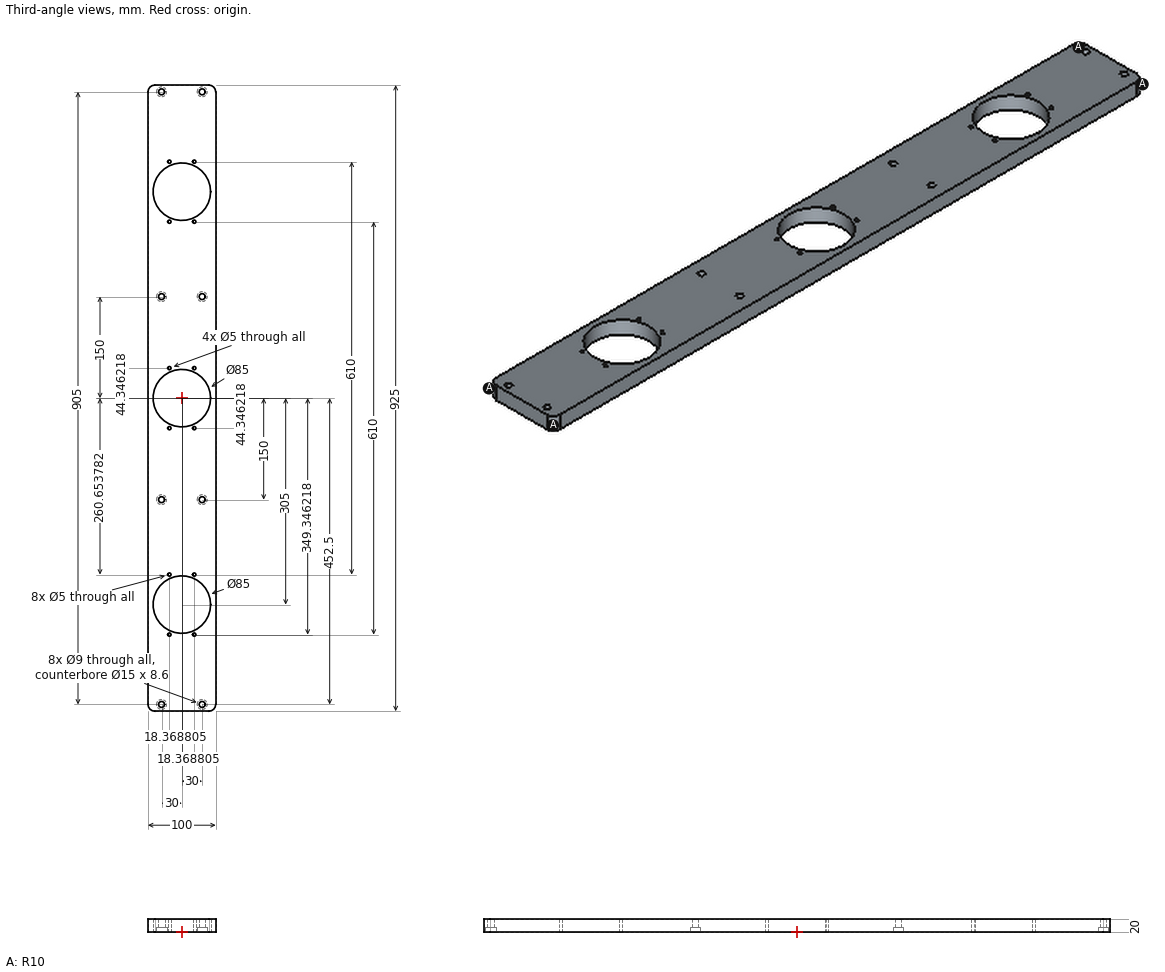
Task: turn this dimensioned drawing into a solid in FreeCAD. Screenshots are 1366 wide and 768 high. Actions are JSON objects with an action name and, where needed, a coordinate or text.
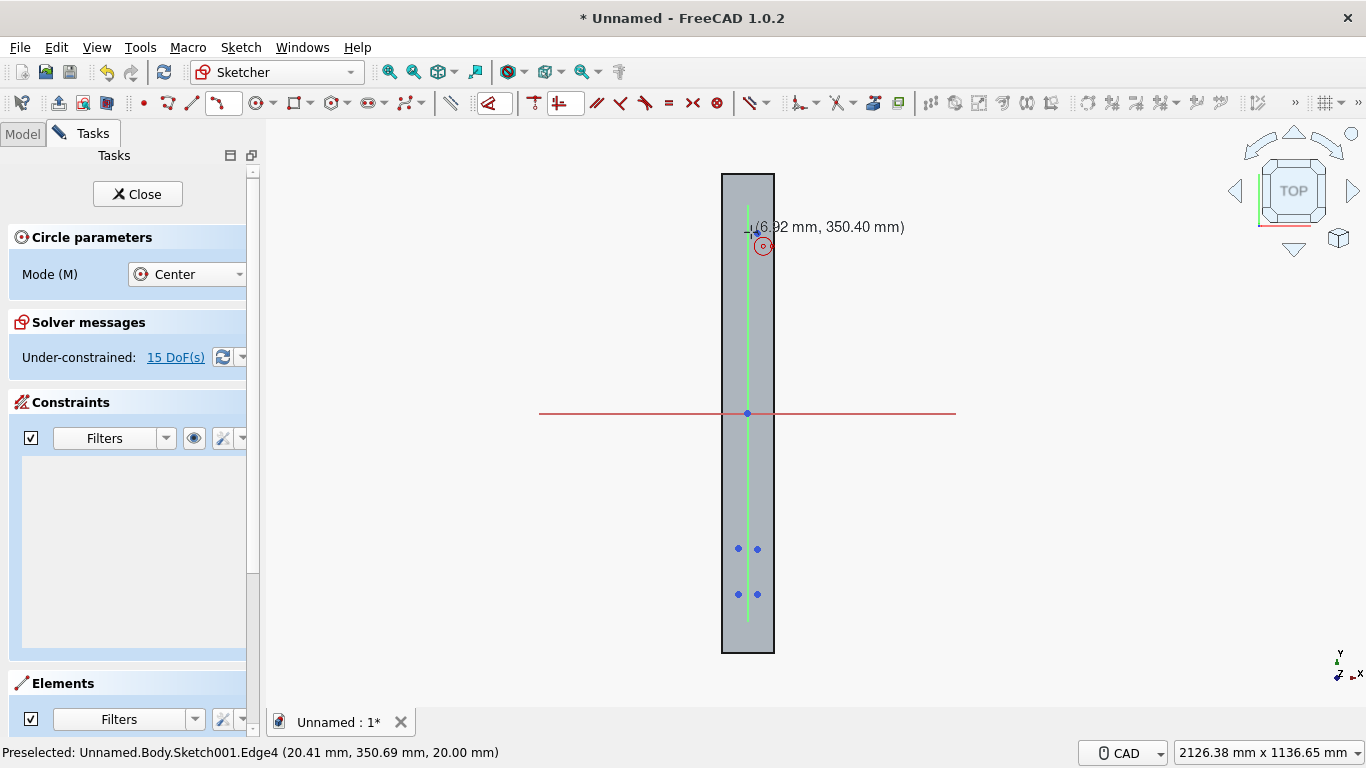
{"action": "scroll", "coordinate": [738, 233], "scroll_direction": "up", "scroll_amount": 3}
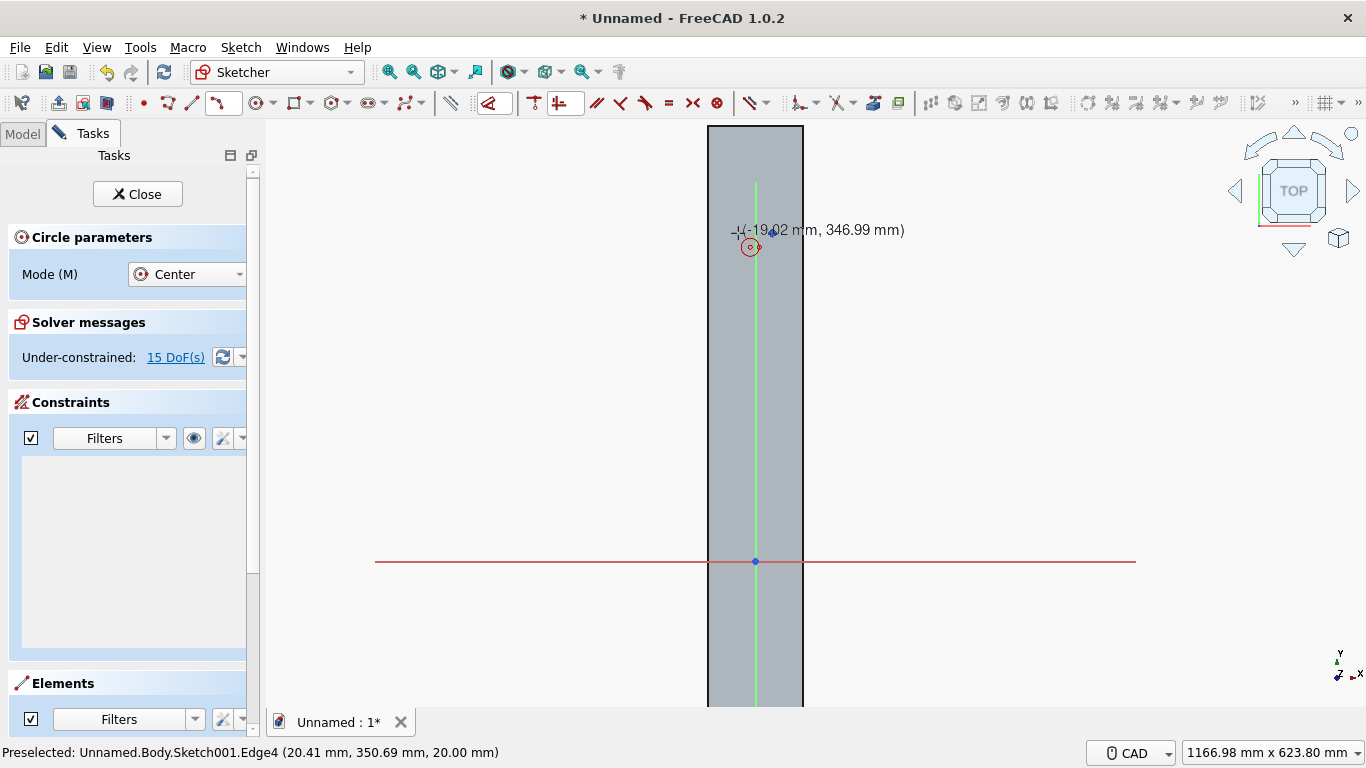
{"action": "left_click", "coordinate": [738, 232]}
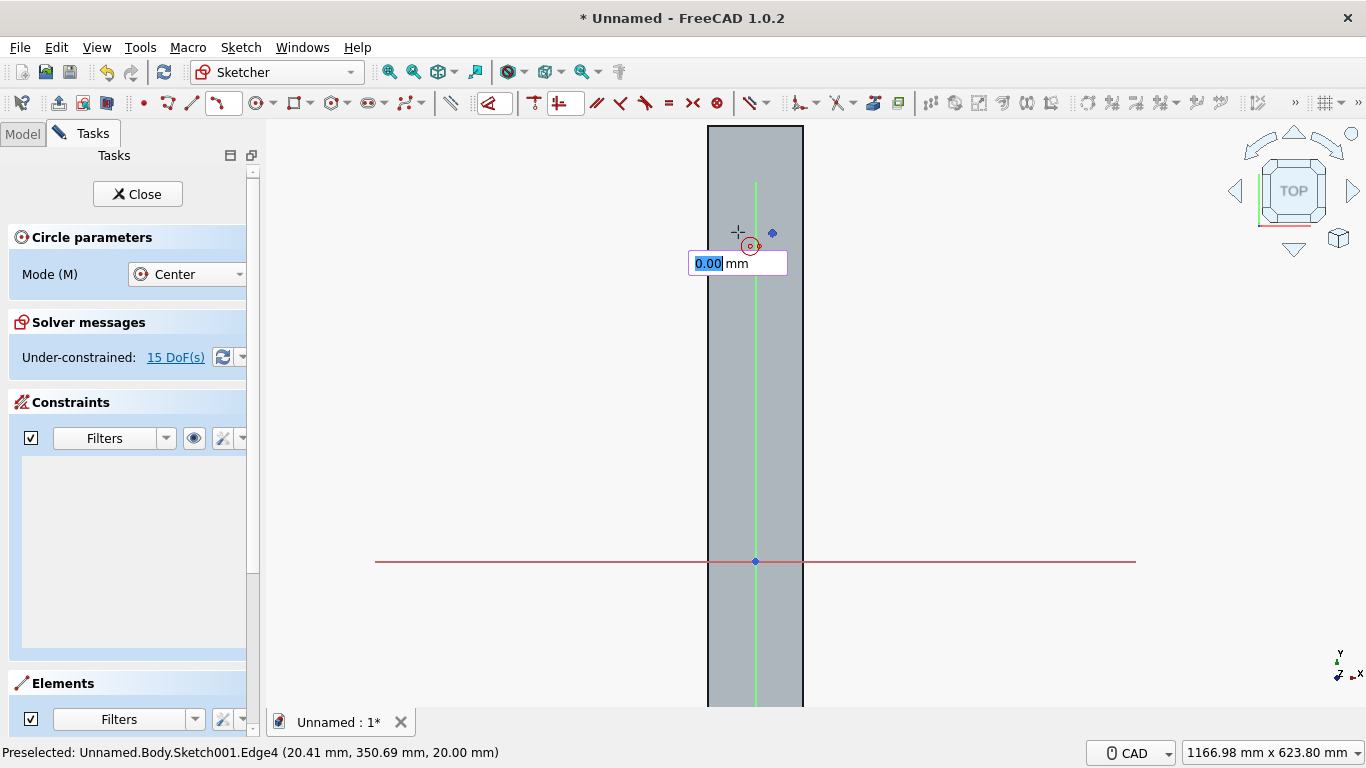
{"action": "scroll", "coordinate": [740, 231], "scroll_direction": "up", "scroll_amount": 10}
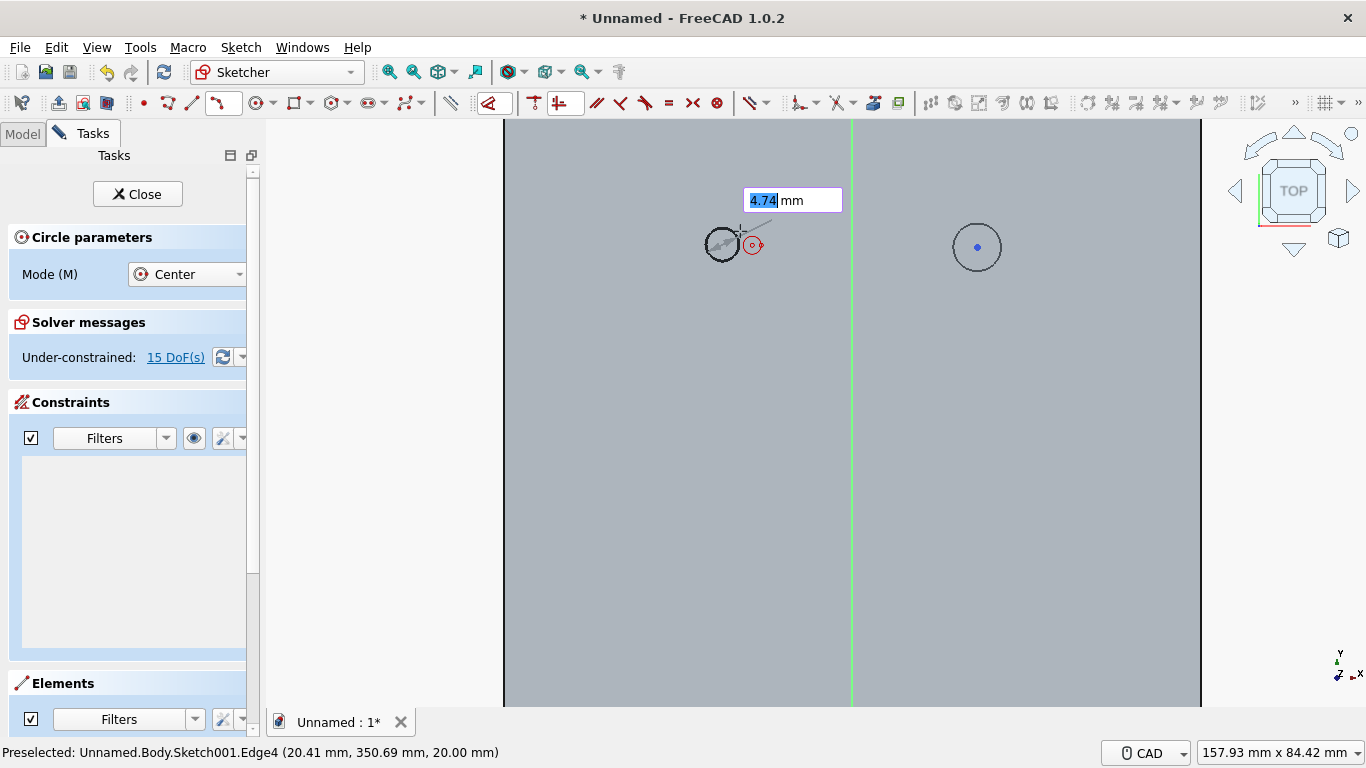
{"action": "left_click", "coordinate": [737, 228]}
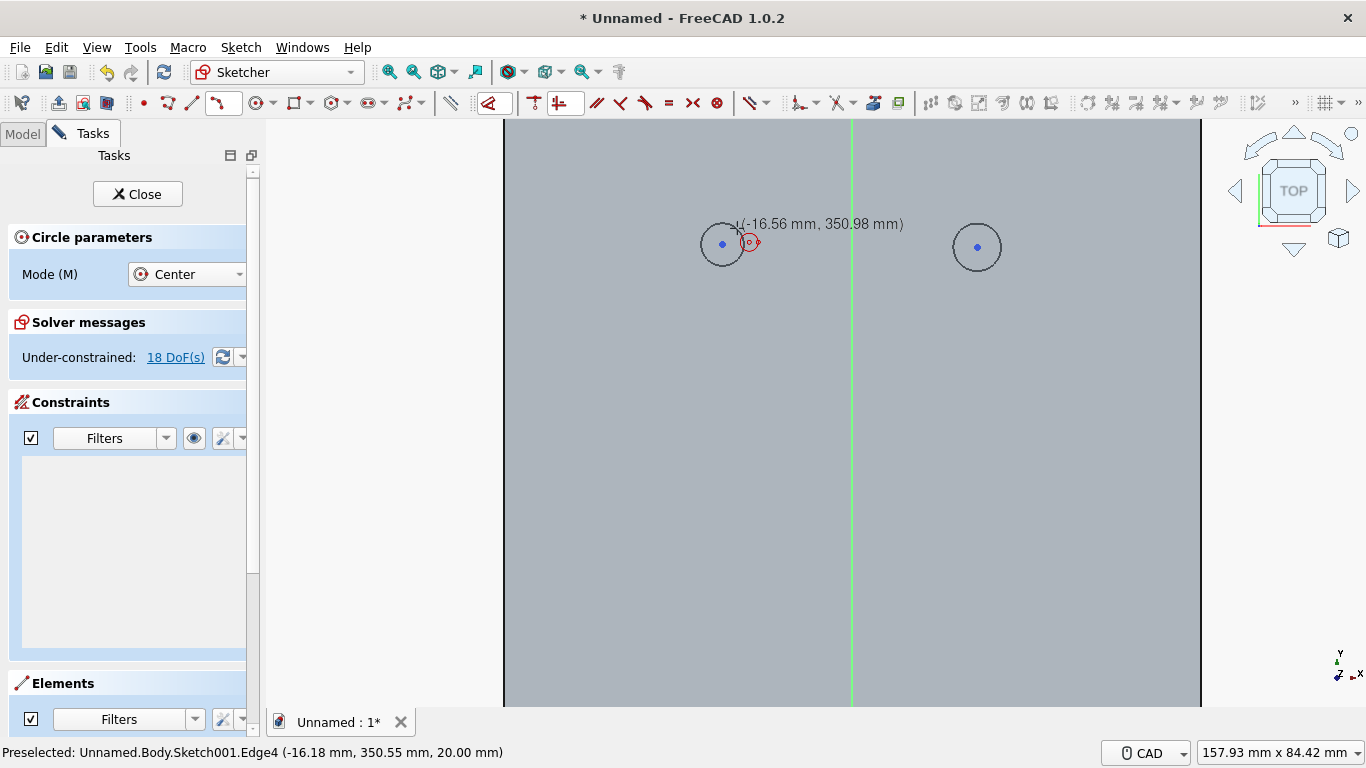
{"action": "scroll", "coordinate": [739, 232], "scroll_direction": "down", "scroll_amount": 13}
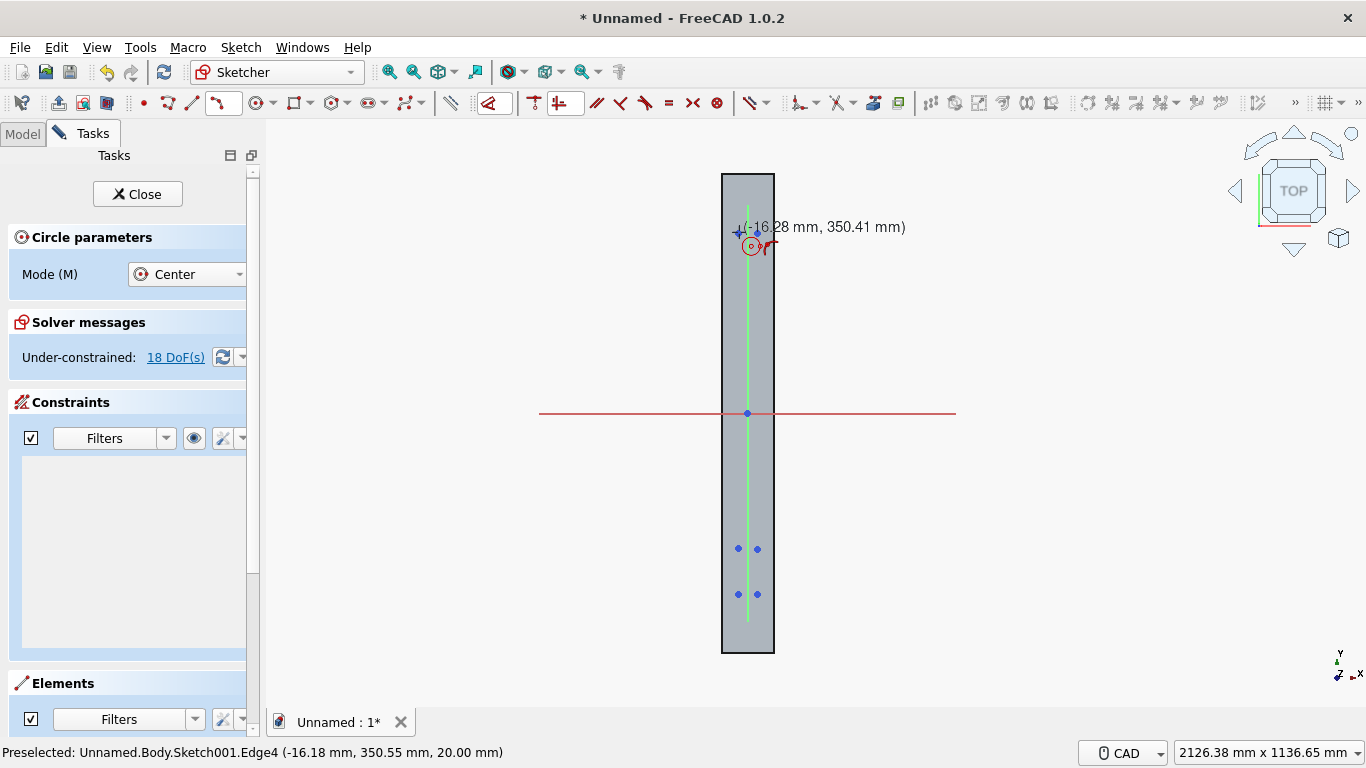
{"action": "scroll", "coordinate": [757, 279], "scroll_direction": "up", "scroll_amount": 15}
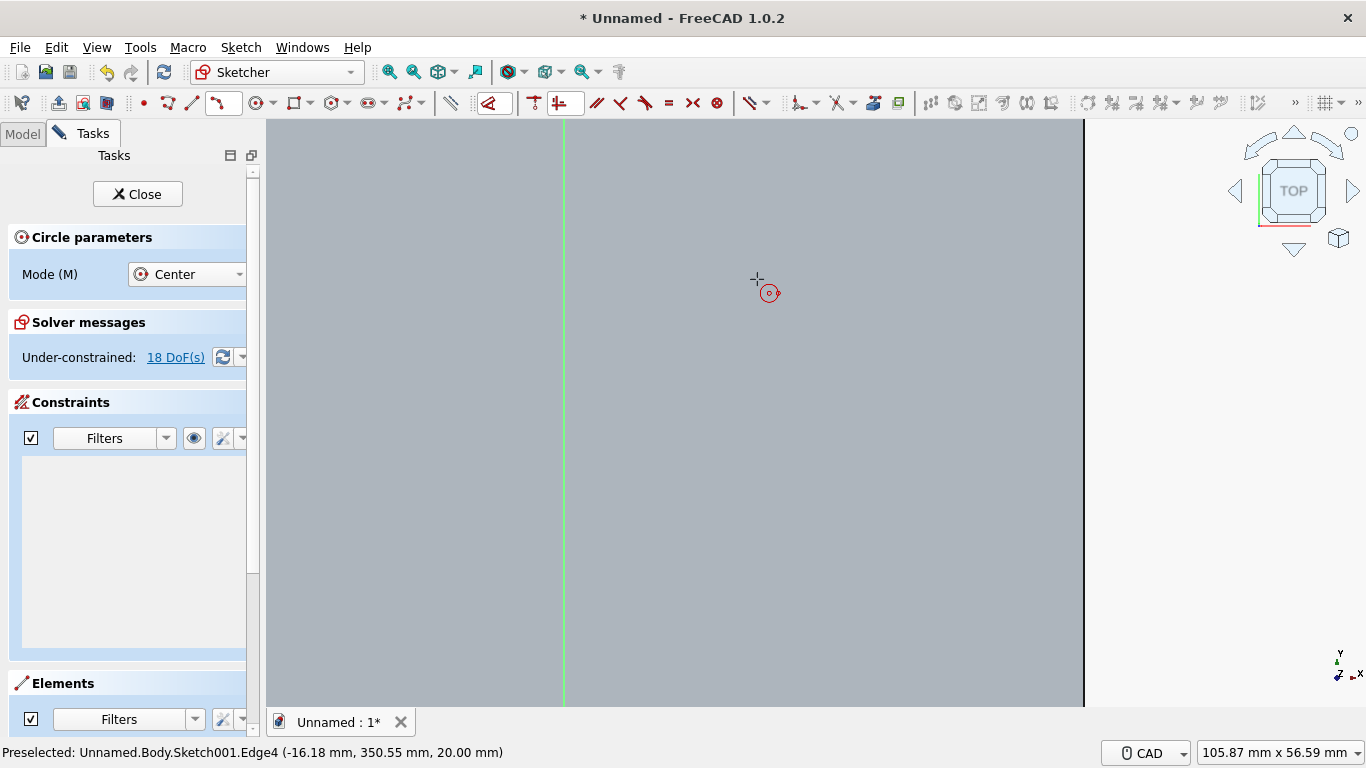
{"action": "scroll", "coordinate": [757, 279], "scroll_direction": "down", "scroll_amount": 15}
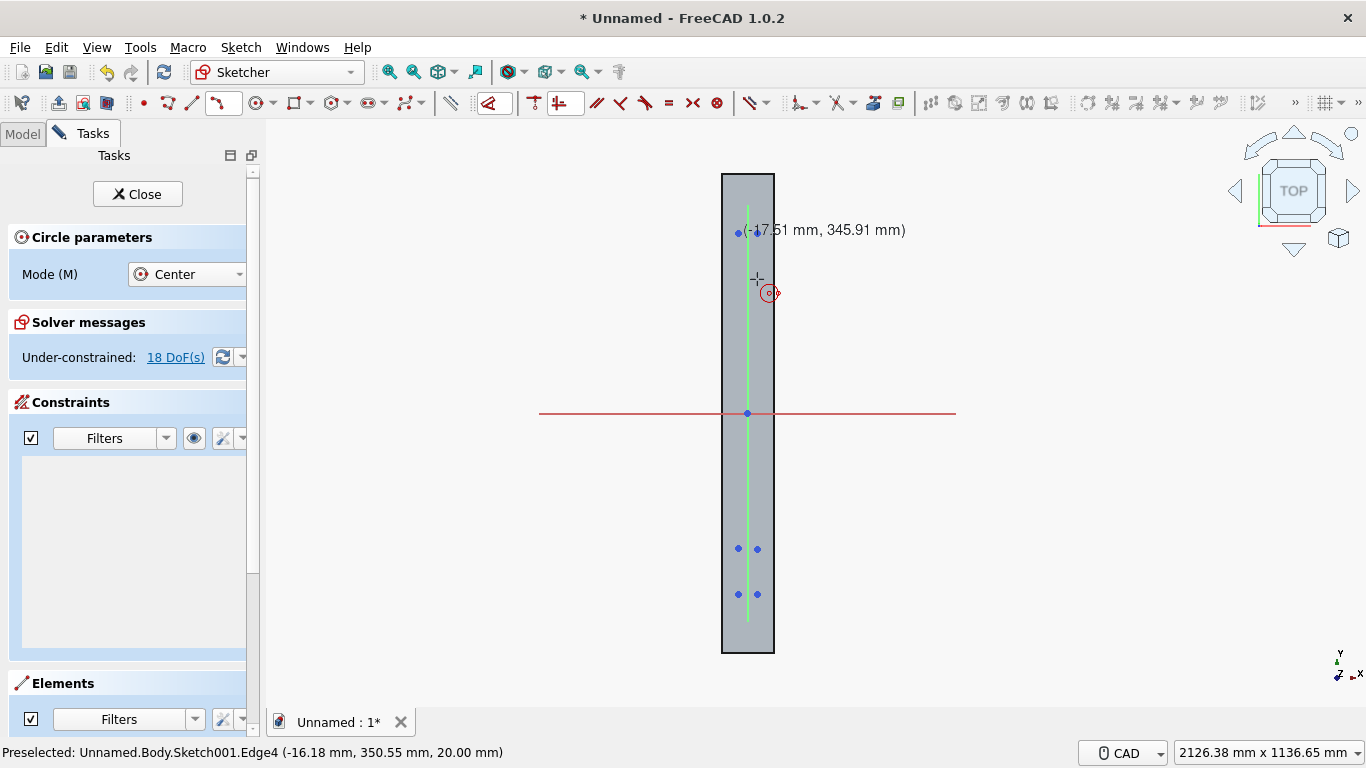
{"action": "scroll", "coordinate": [757, 279], "scroll_direction": "up", "scroll_amount": 3}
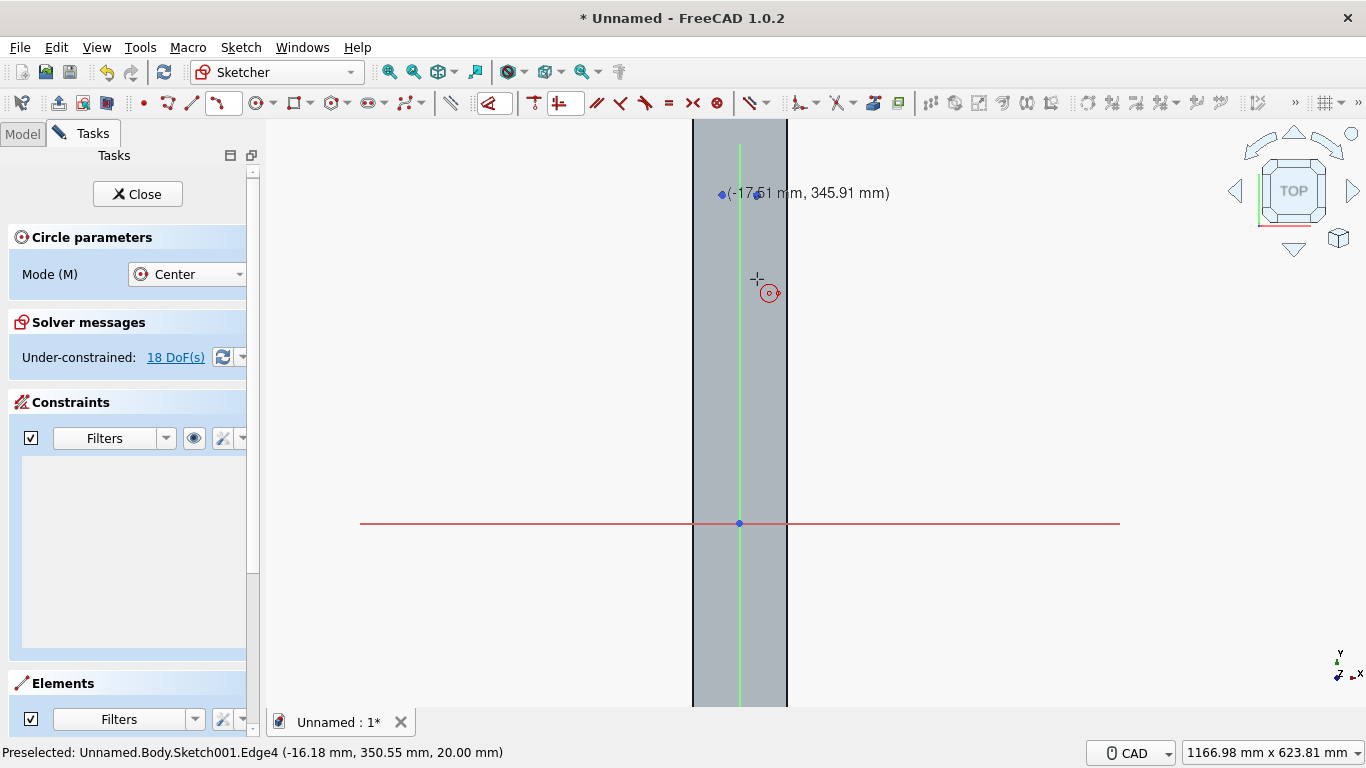
{"action": "left_click", "coordinate": [757, 278]}